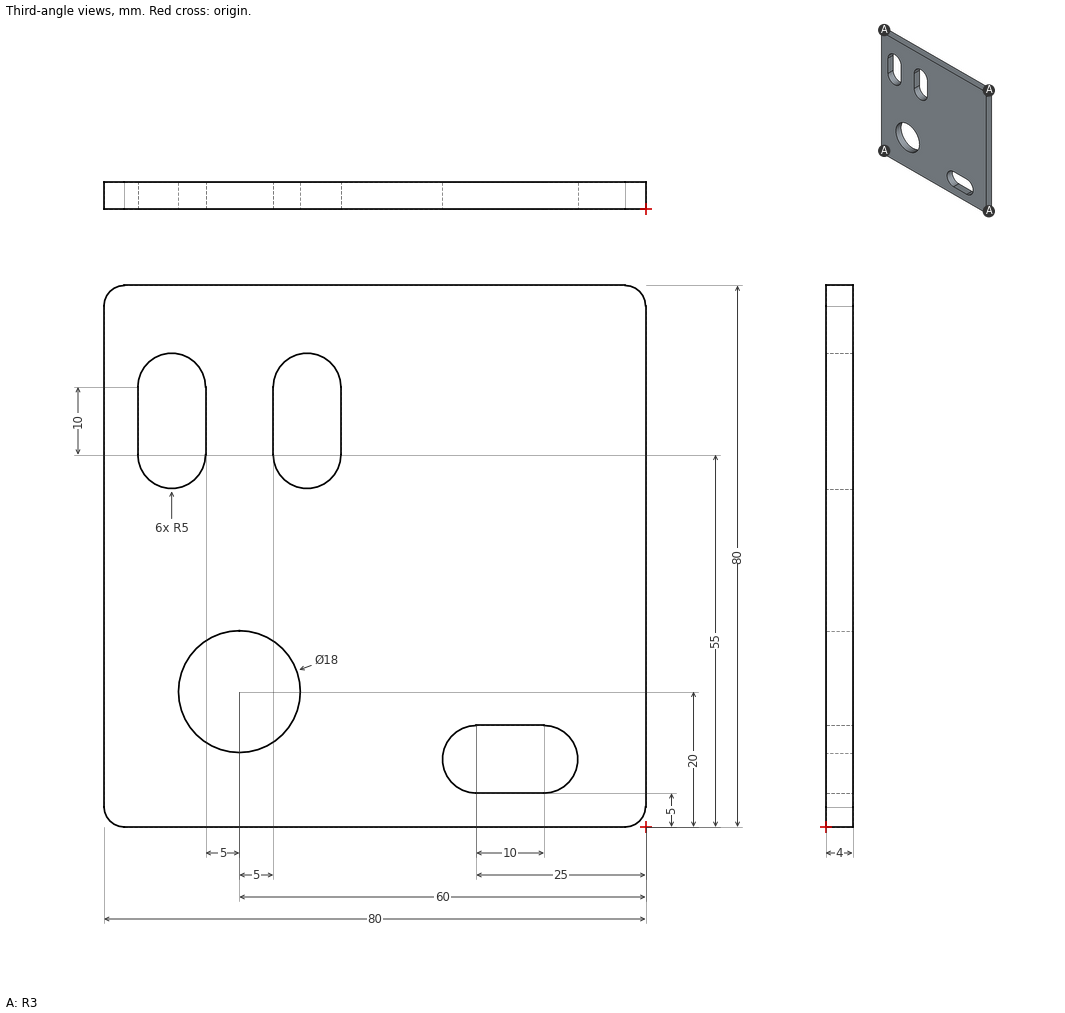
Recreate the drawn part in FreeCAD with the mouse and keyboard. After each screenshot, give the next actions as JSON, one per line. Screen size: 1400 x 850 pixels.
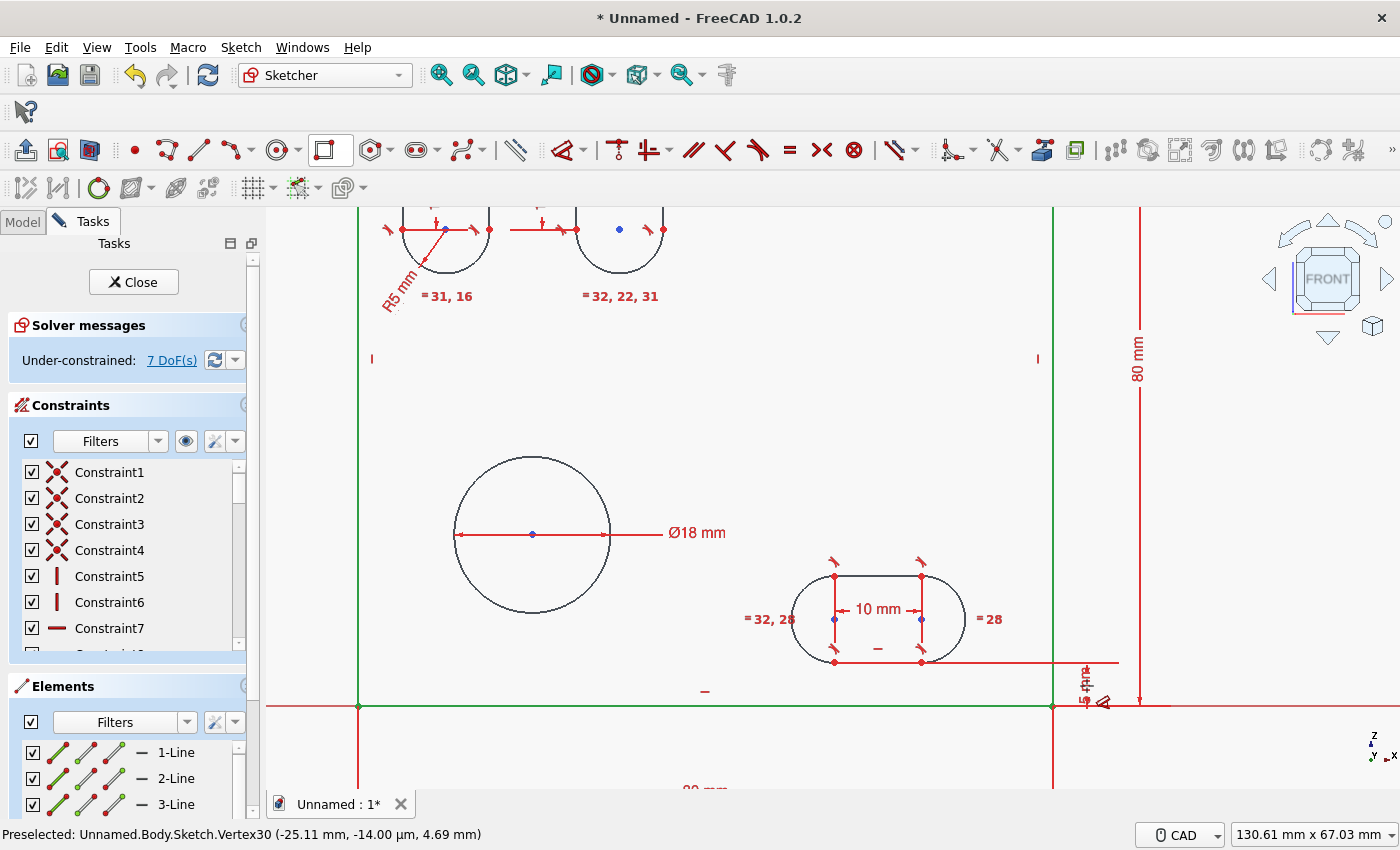
{"action": "left_click", "coordinate": [532, 535]}
{"action": "left_click", "coordinate": [793, 740]}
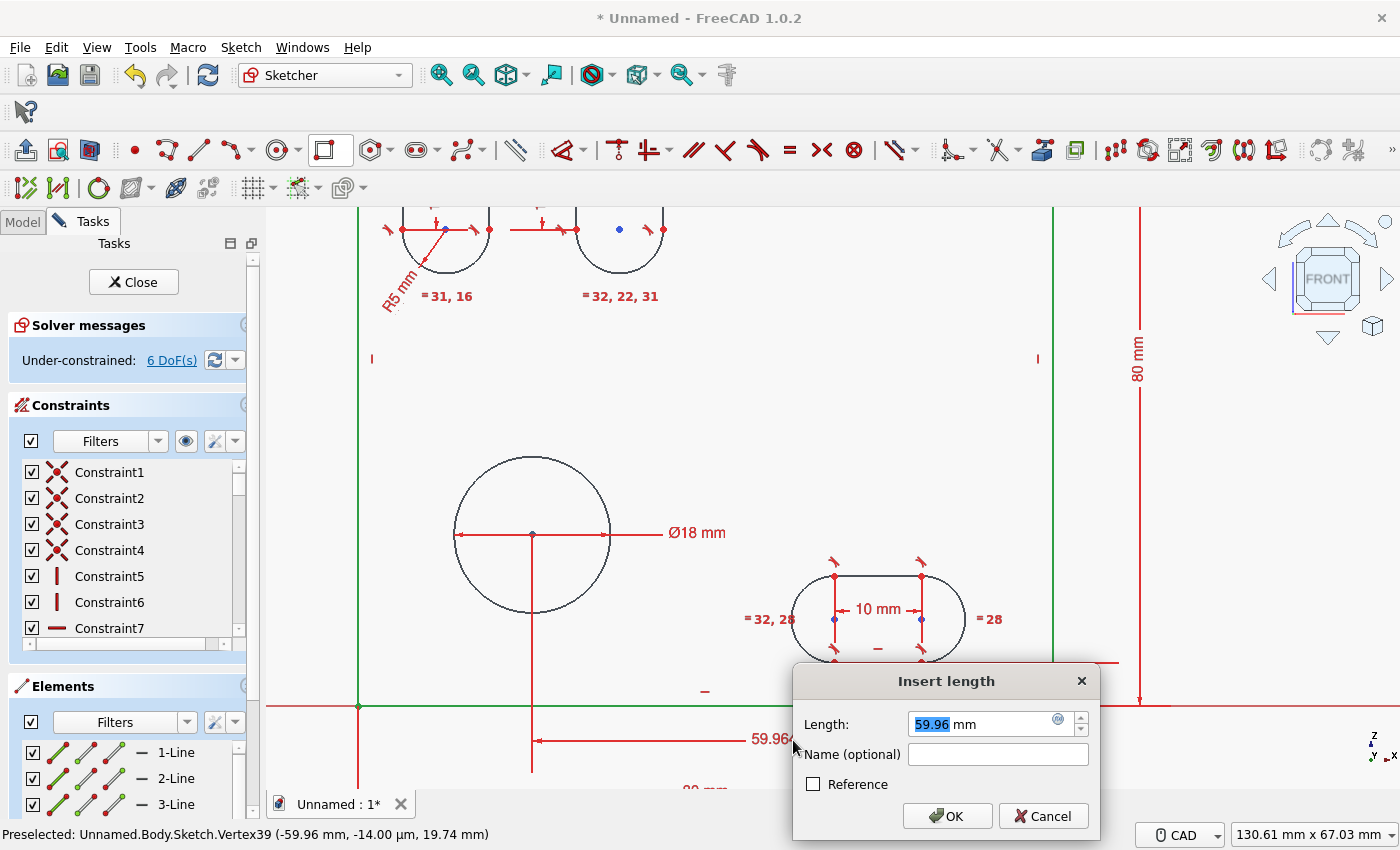
{"action": "type", "text": "60"}
{"action": "key", "text": "Return"}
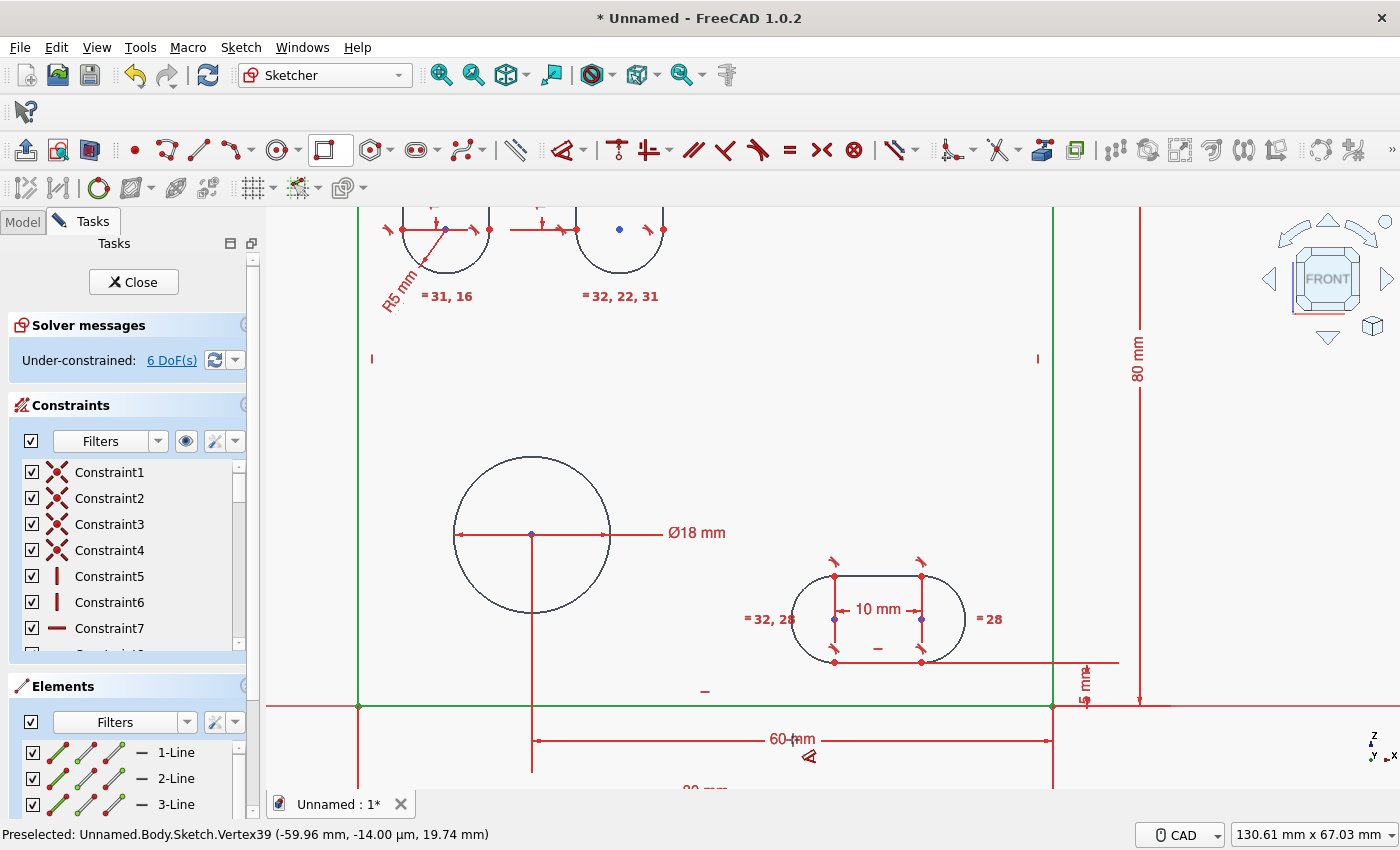
{"action": "left_click", "coordinate": [532, 535]}
{"action": "left_click", "coordinate": [1087, 621]}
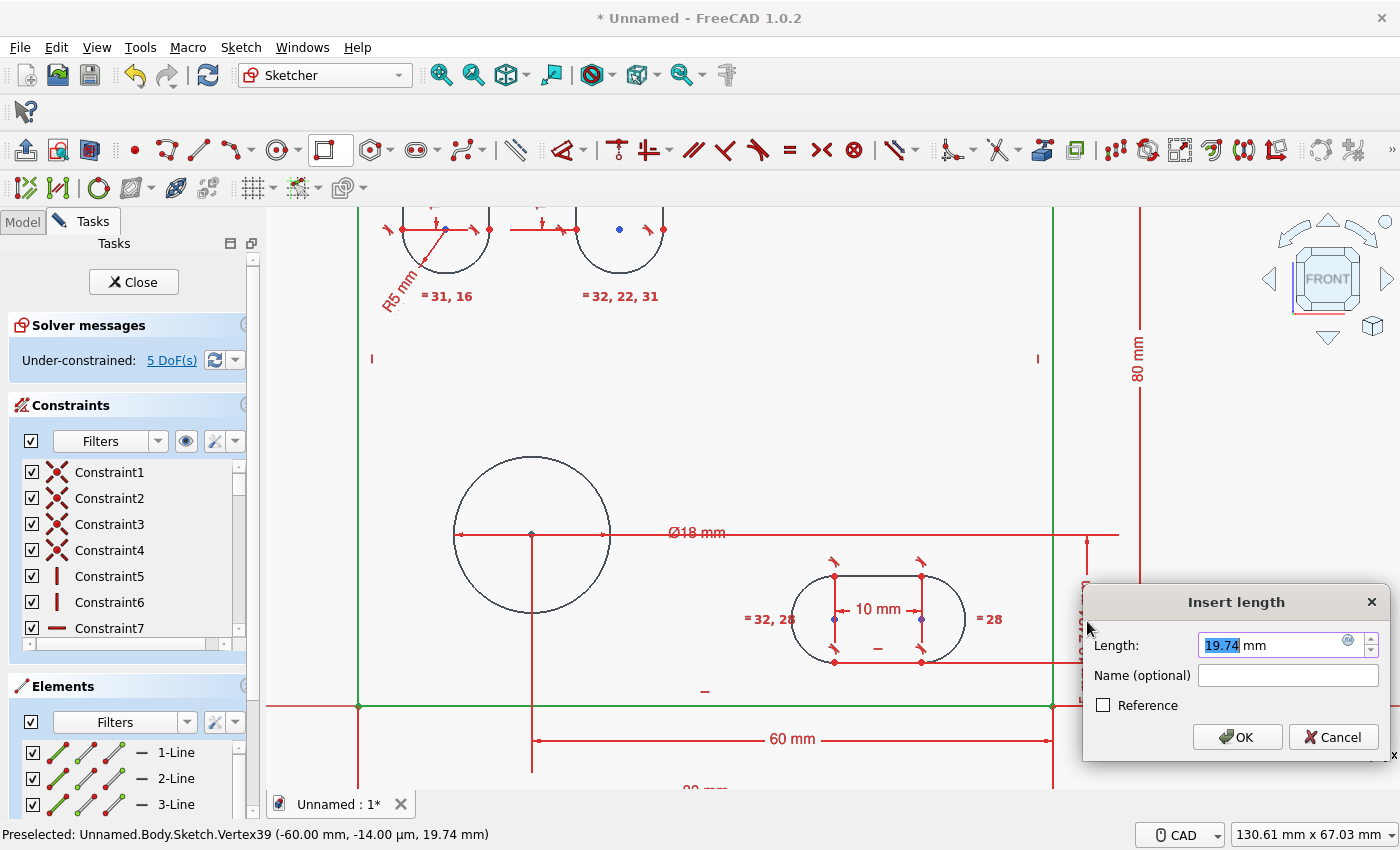
{"action": "type", "text": "20"}
{"action": "key", "text": "Return"}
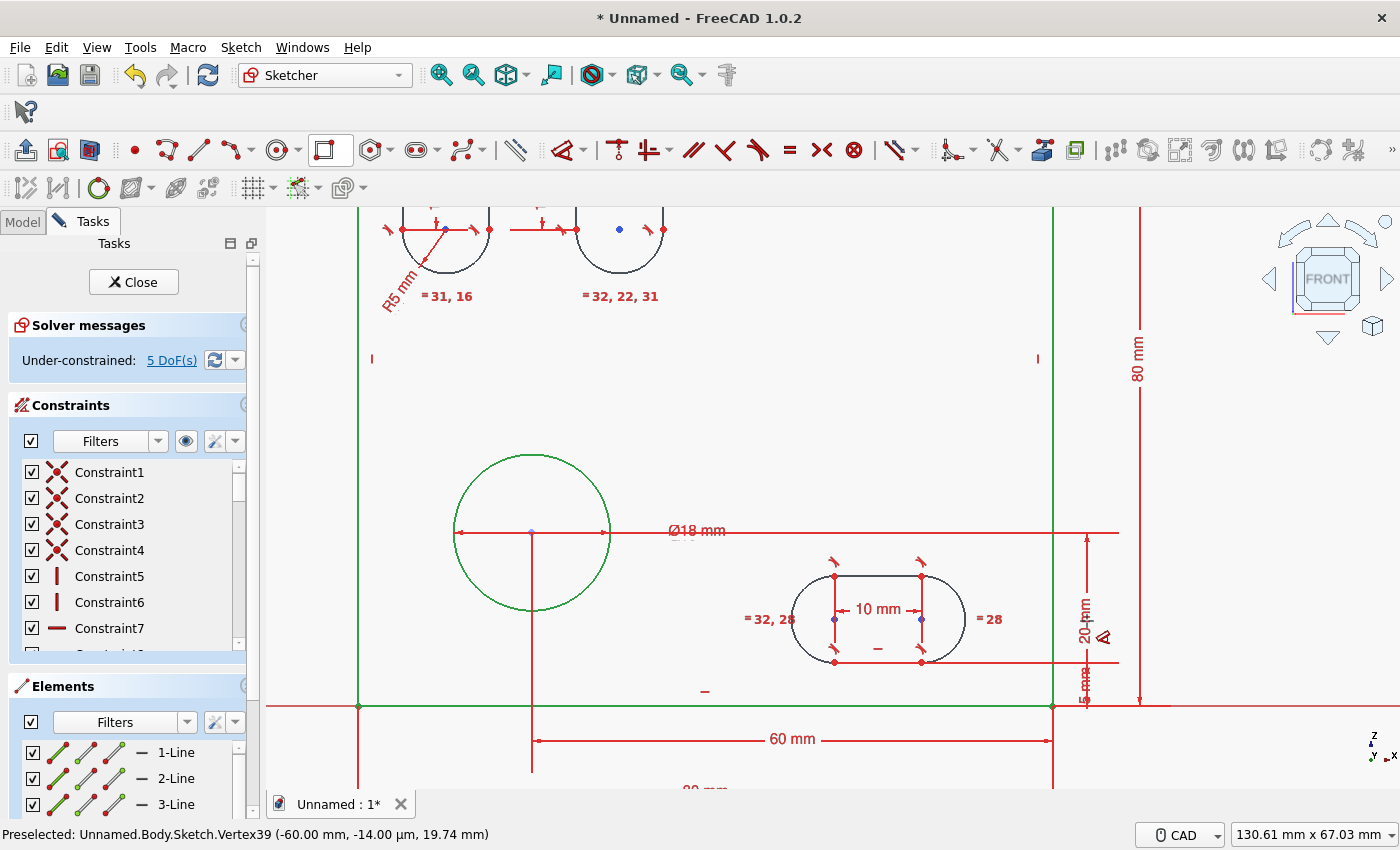
{"action": "scroll", "coordinate": [836, 667], "scroll_direction": "down", "scroll_amount": 3}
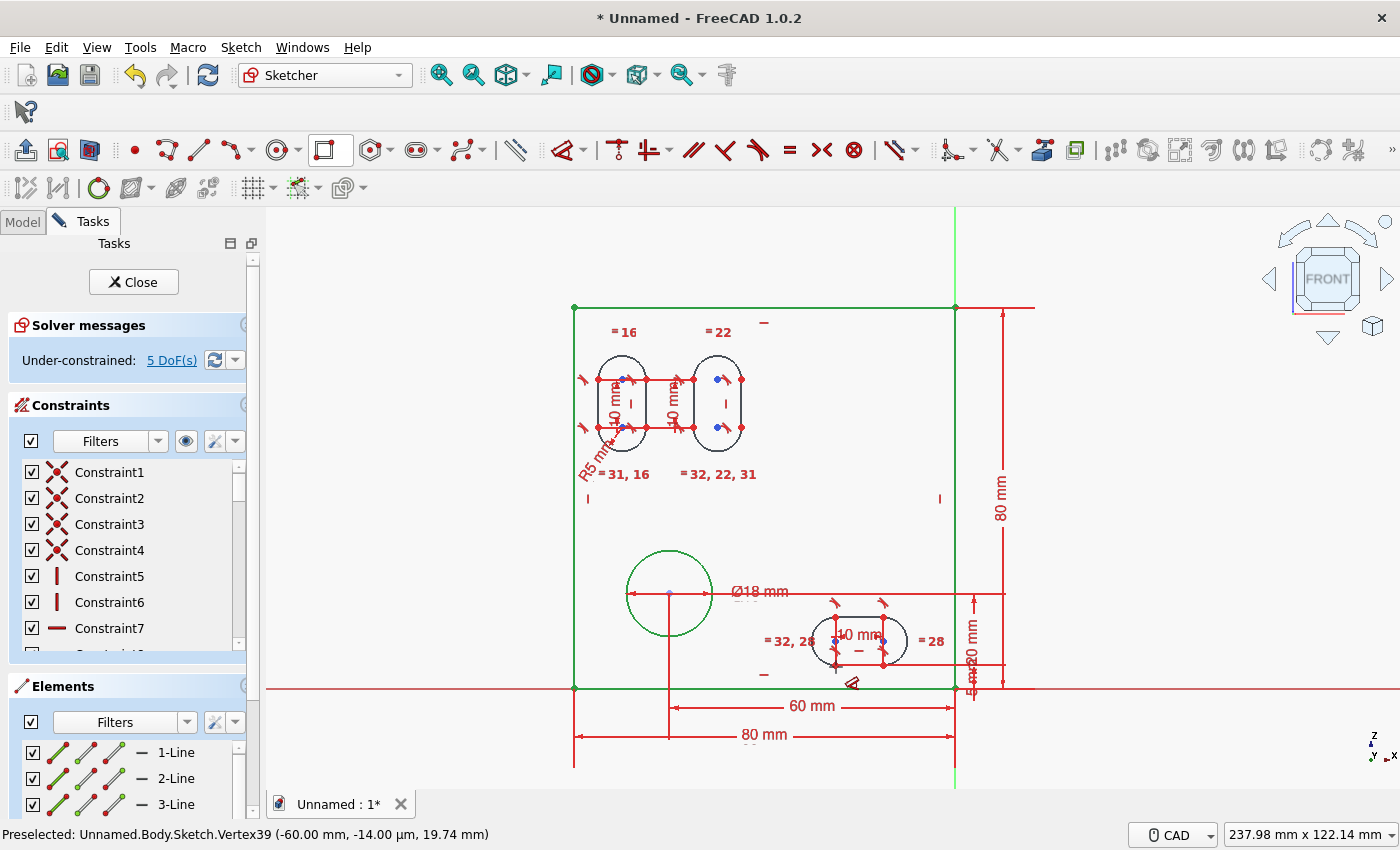
{"action": "scroll", "coordinate": [646, 428], "scroll_direction": "up", "scroll_amount": 3}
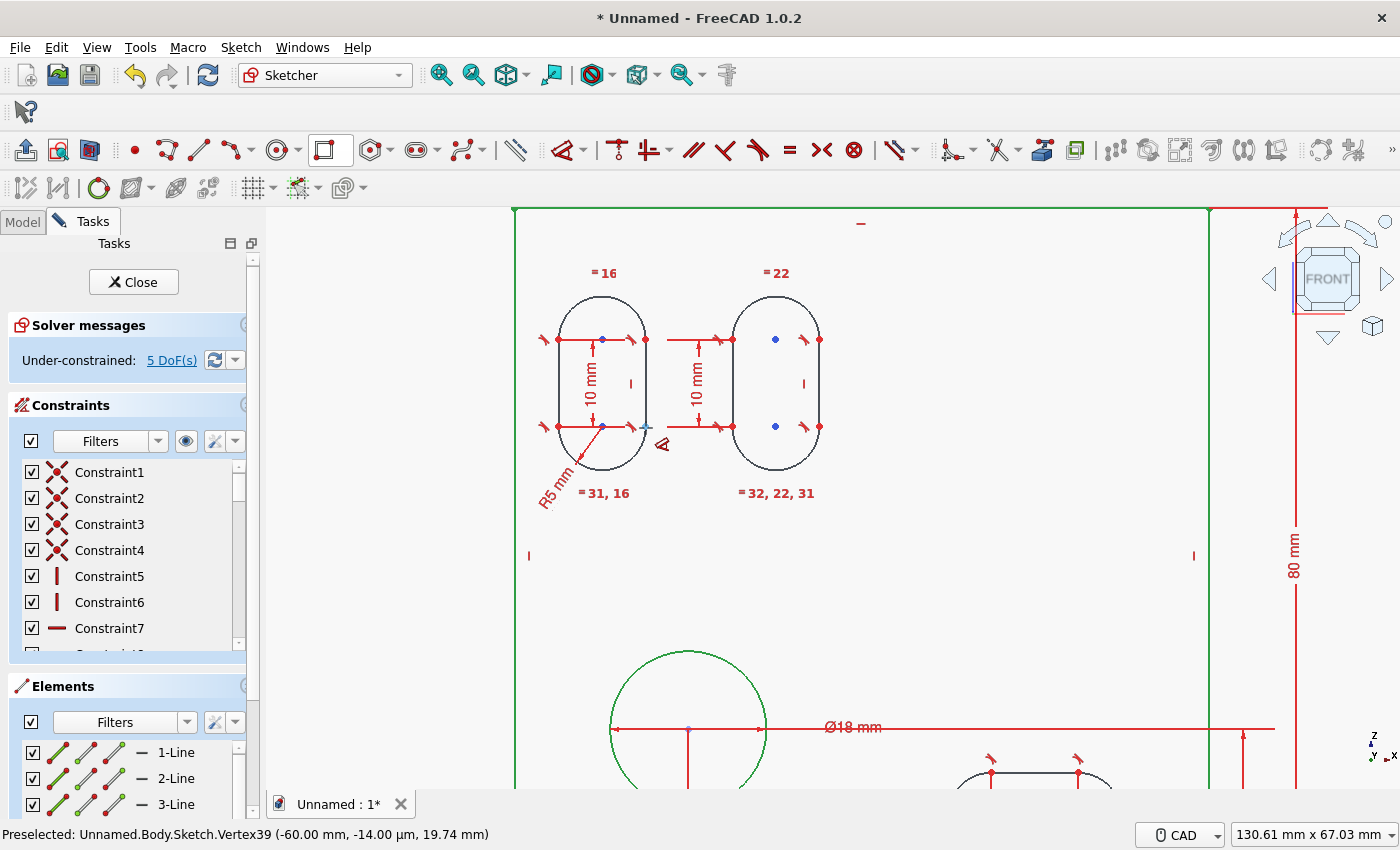
{"action": "left_click", "coordinate": [646, 427]}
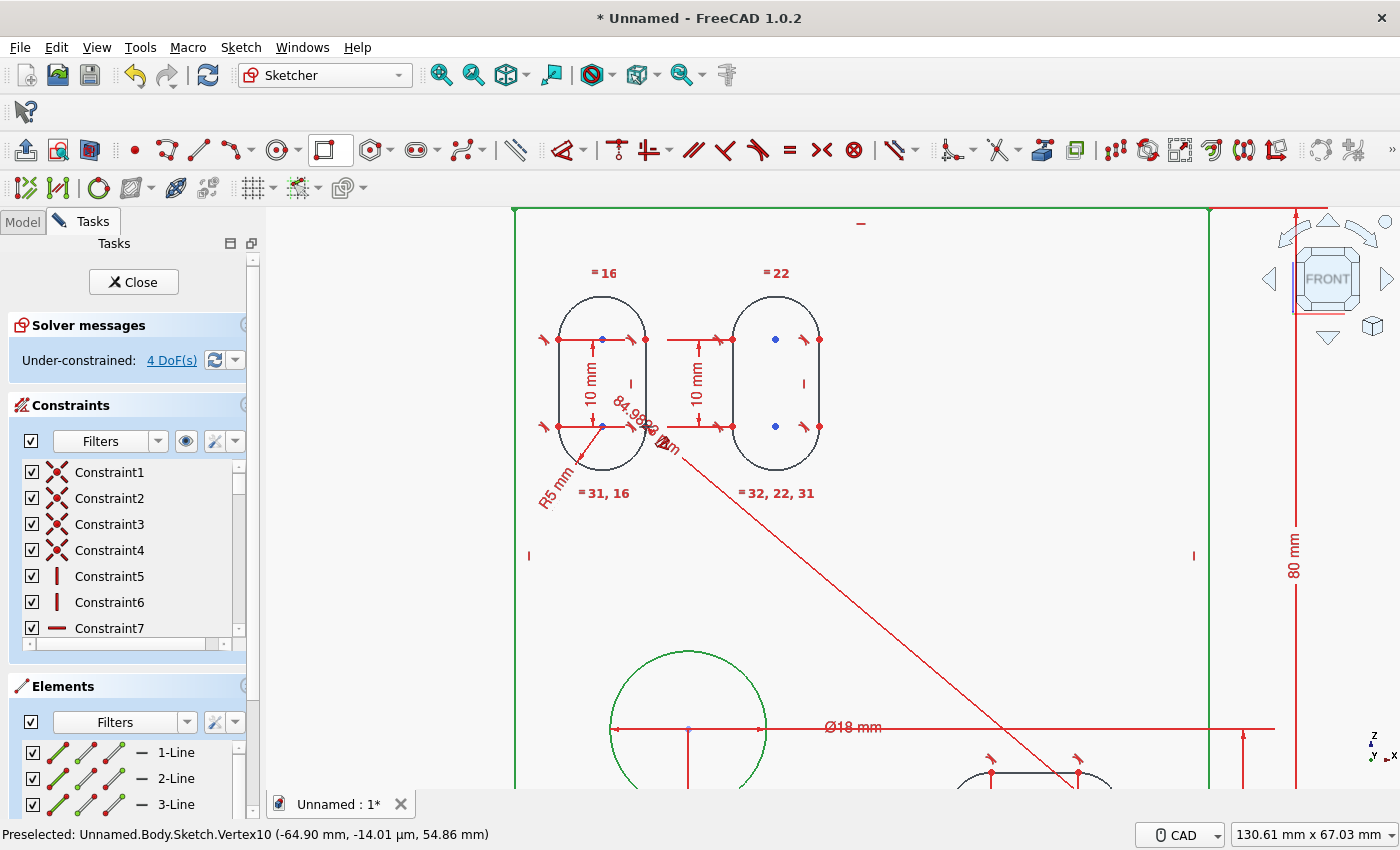
{"action": "left_click", "coordinate": [688, 729]}
{"action": "left_click", "coordinate": [667, 345]}